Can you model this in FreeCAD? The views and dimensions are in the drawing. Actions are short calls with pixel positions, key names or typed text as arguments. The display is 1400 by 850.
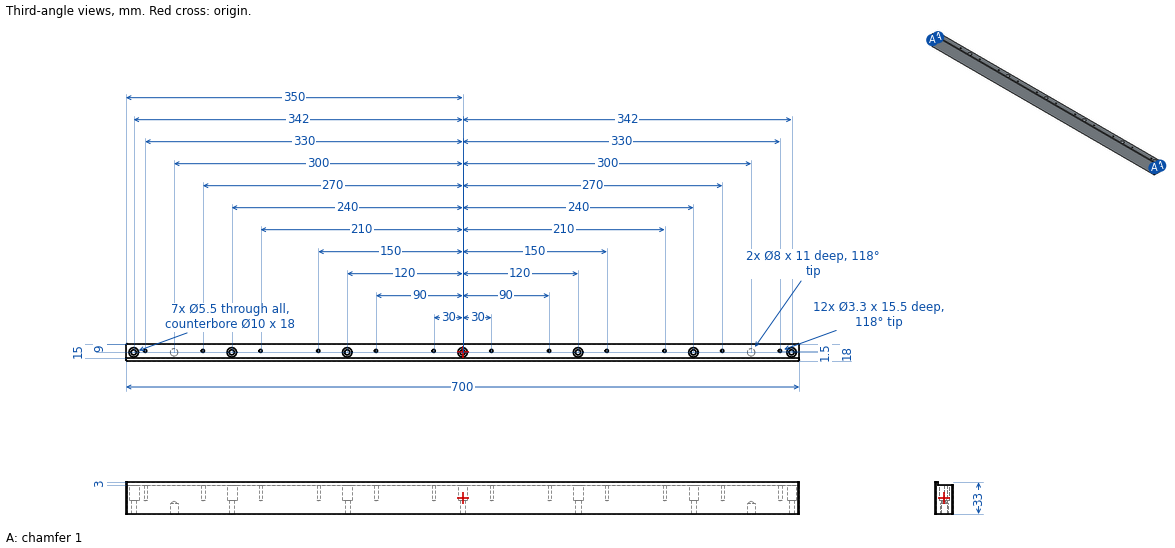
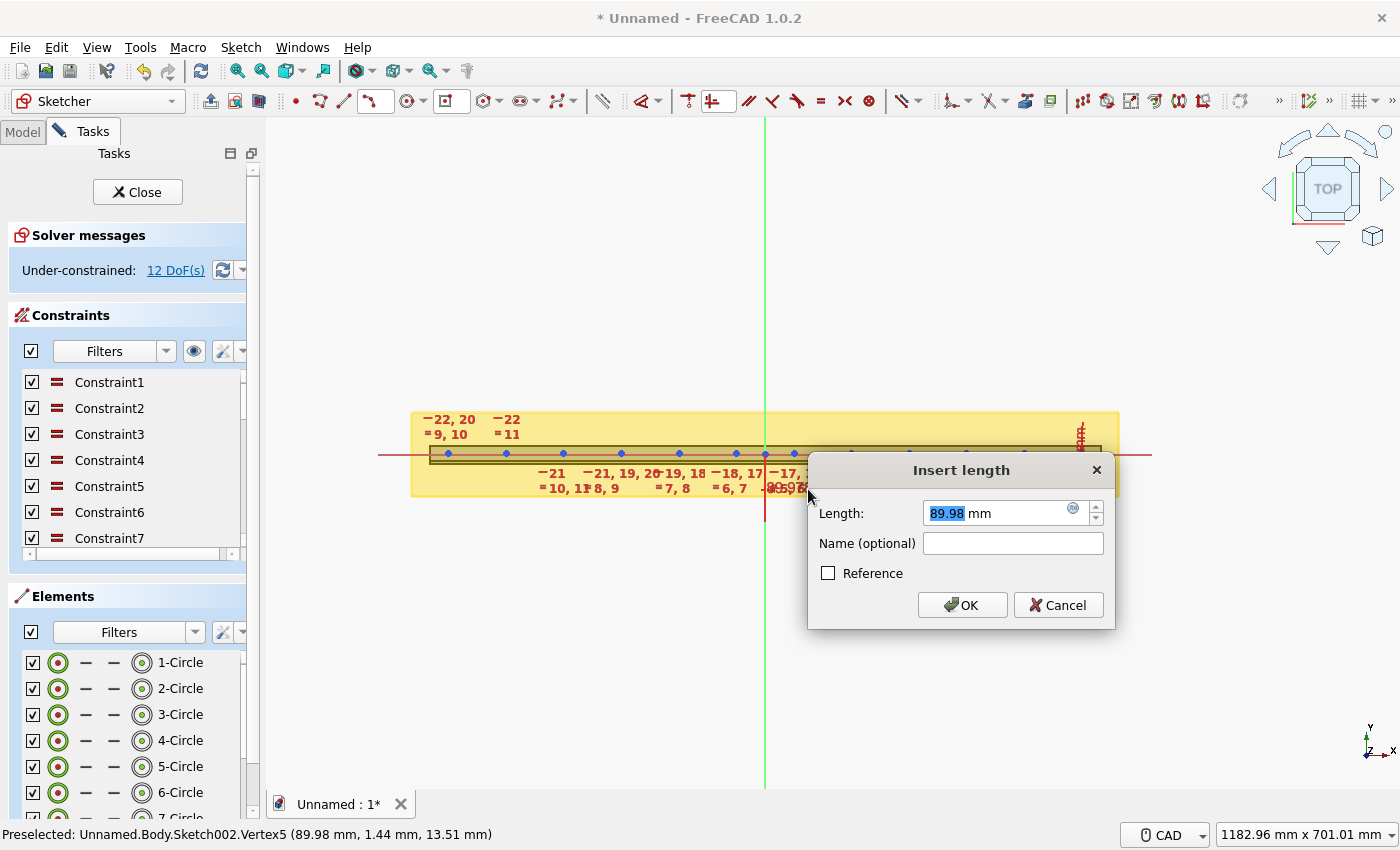
text(90)
key(Return)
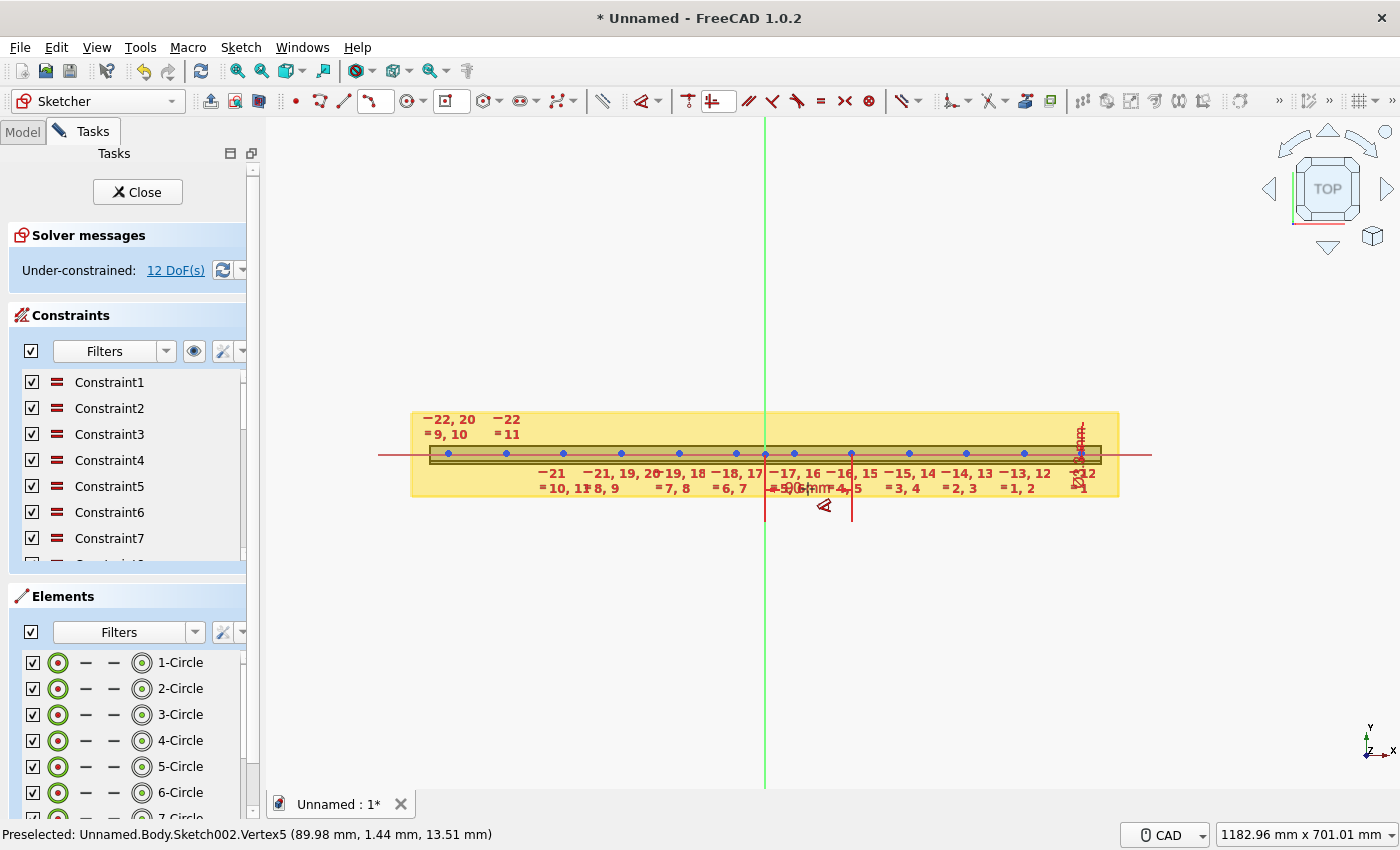
scroll(794, 453, up, 2)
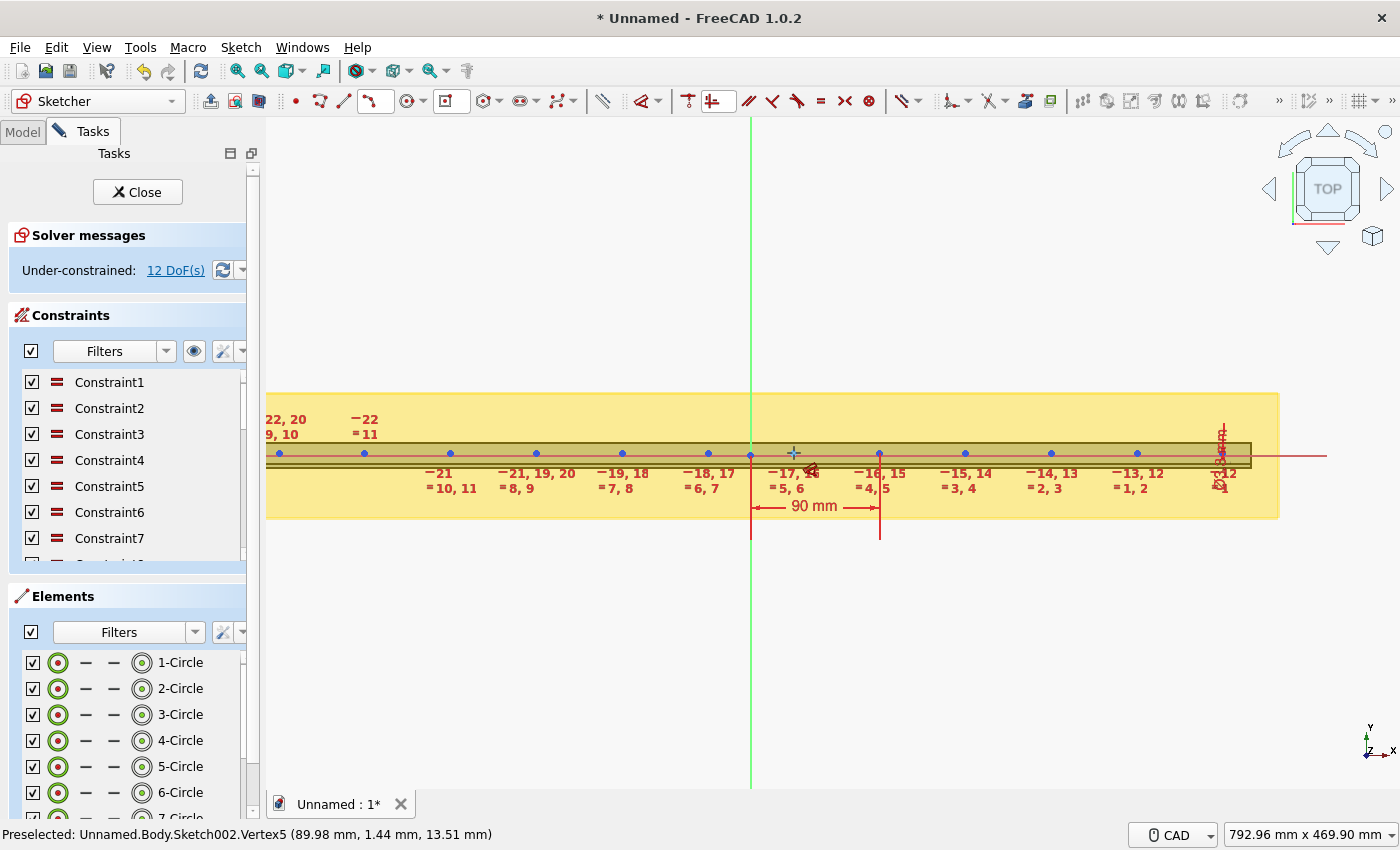
click(794, 453)
click(772, 419)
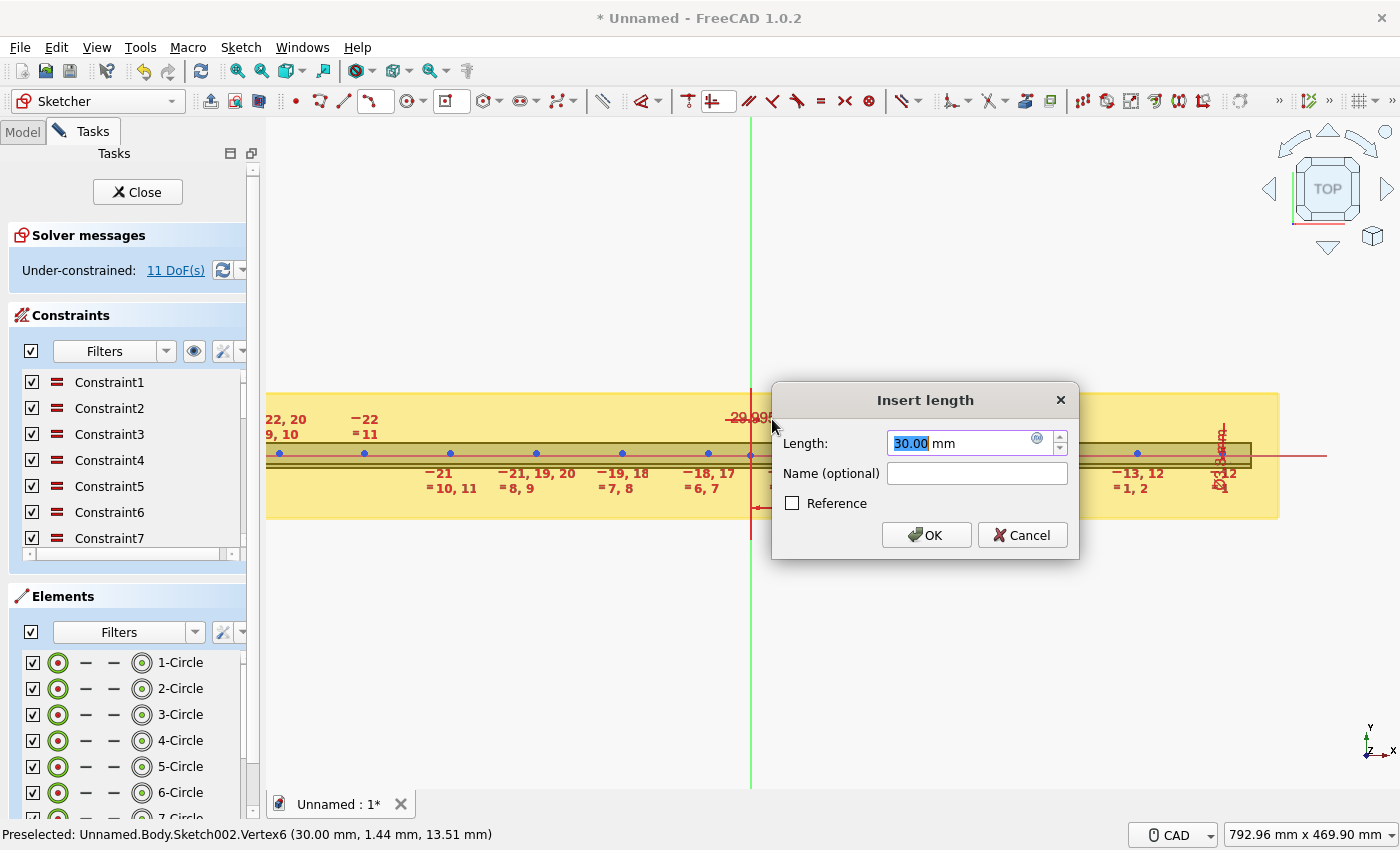
text(30)
key(Return)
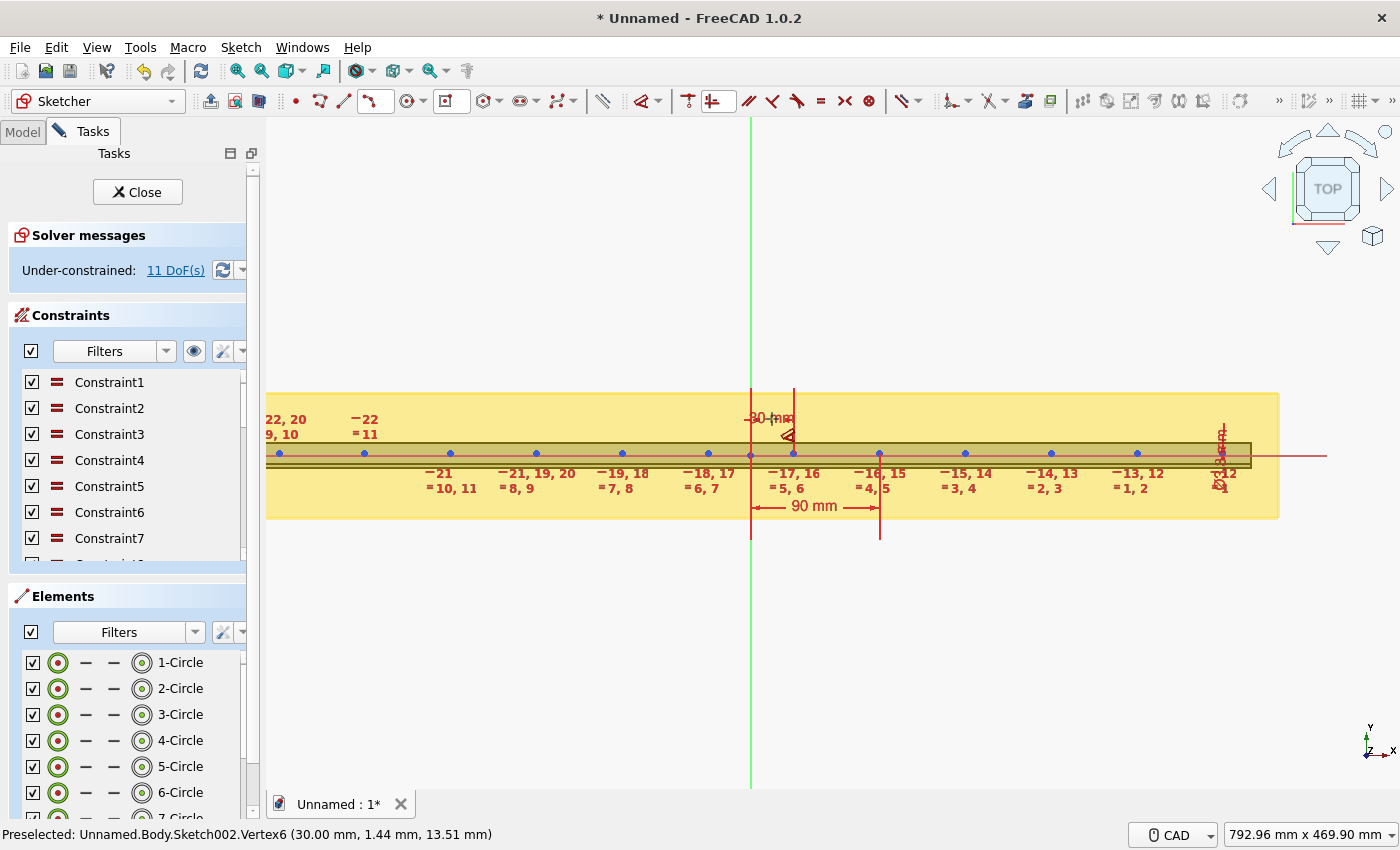
click(708, 453)
click(729, 490)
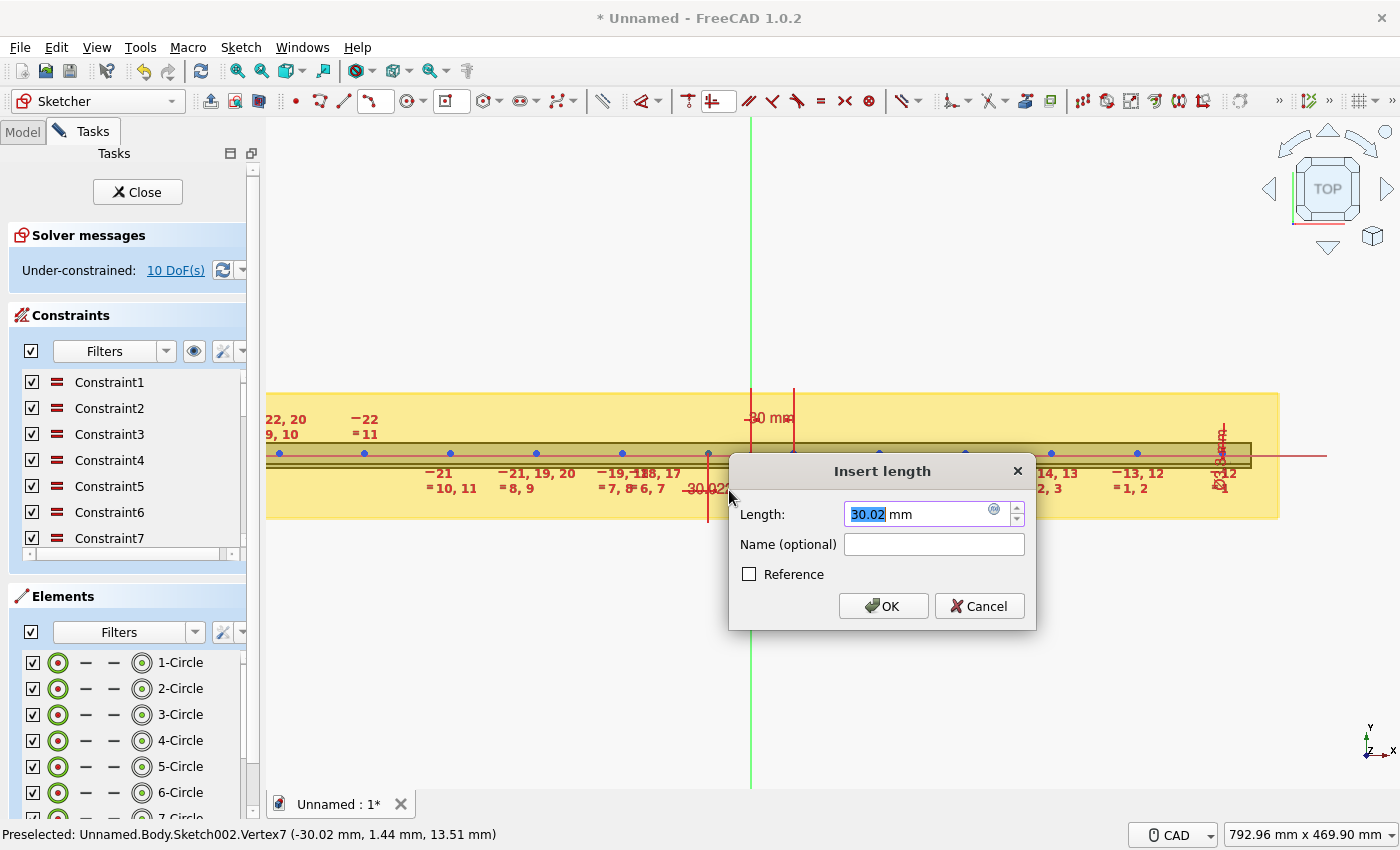
text(30)
key(Return)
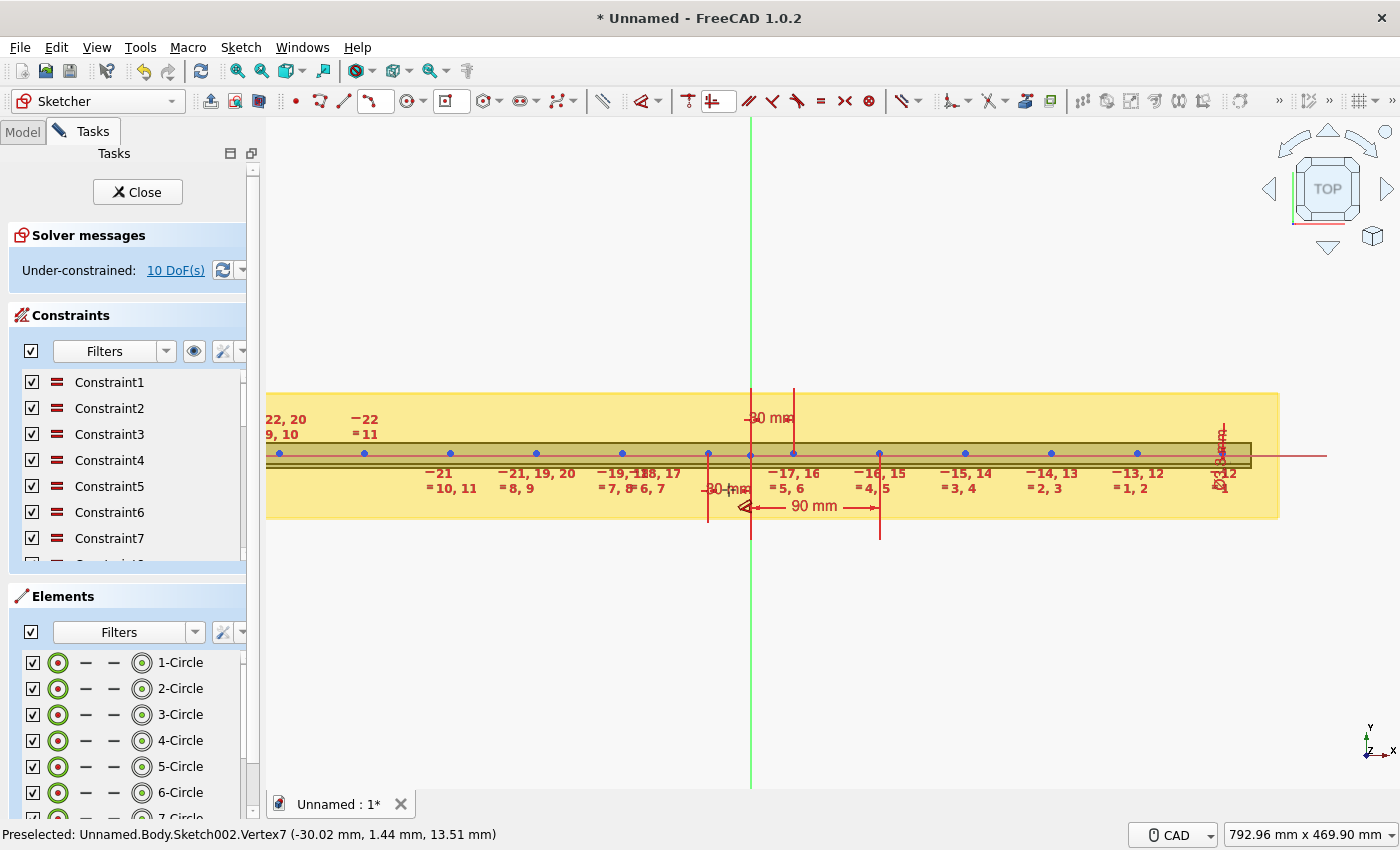
click(622, 453)
click(657, 490)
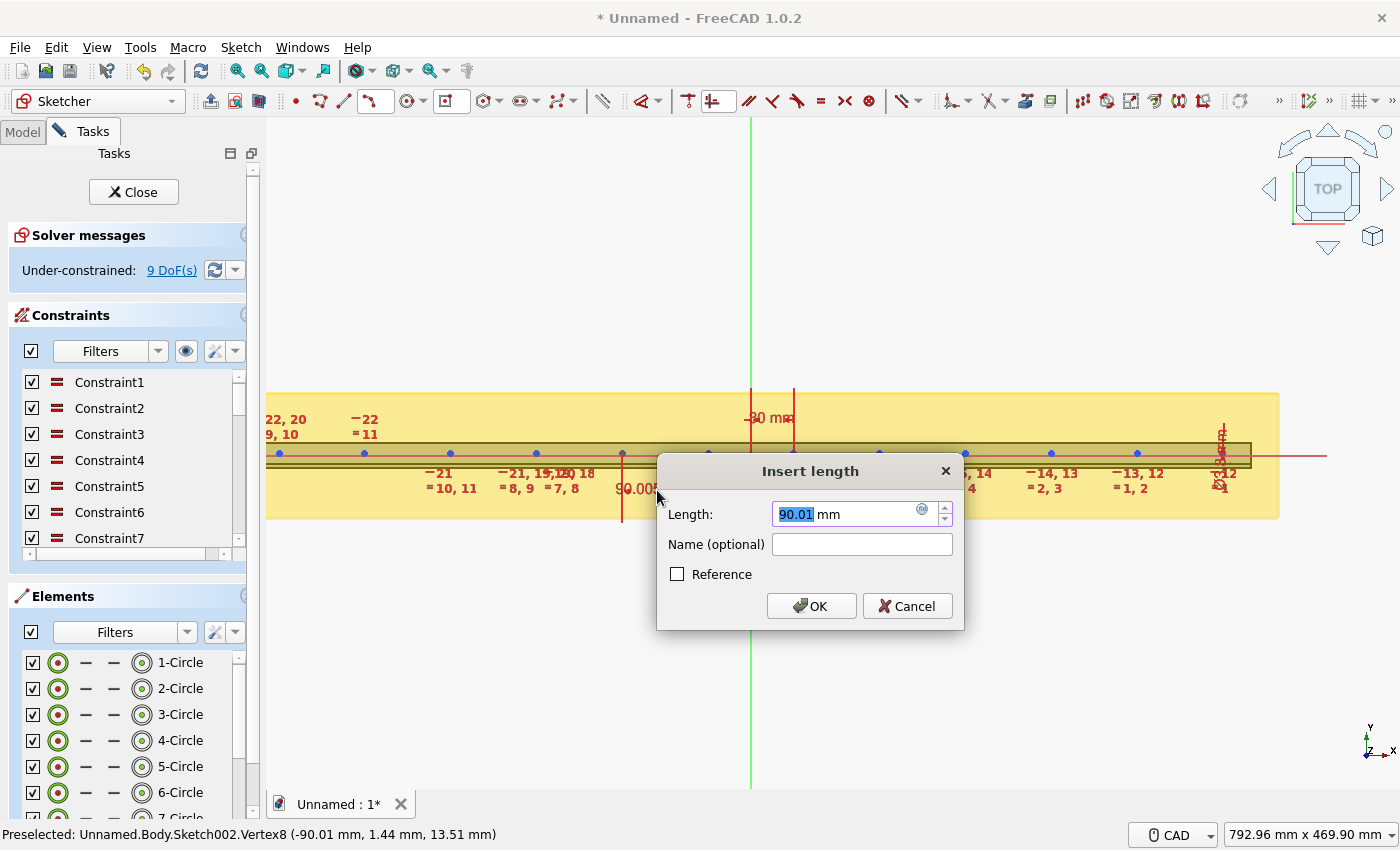
text(90)
key(Return)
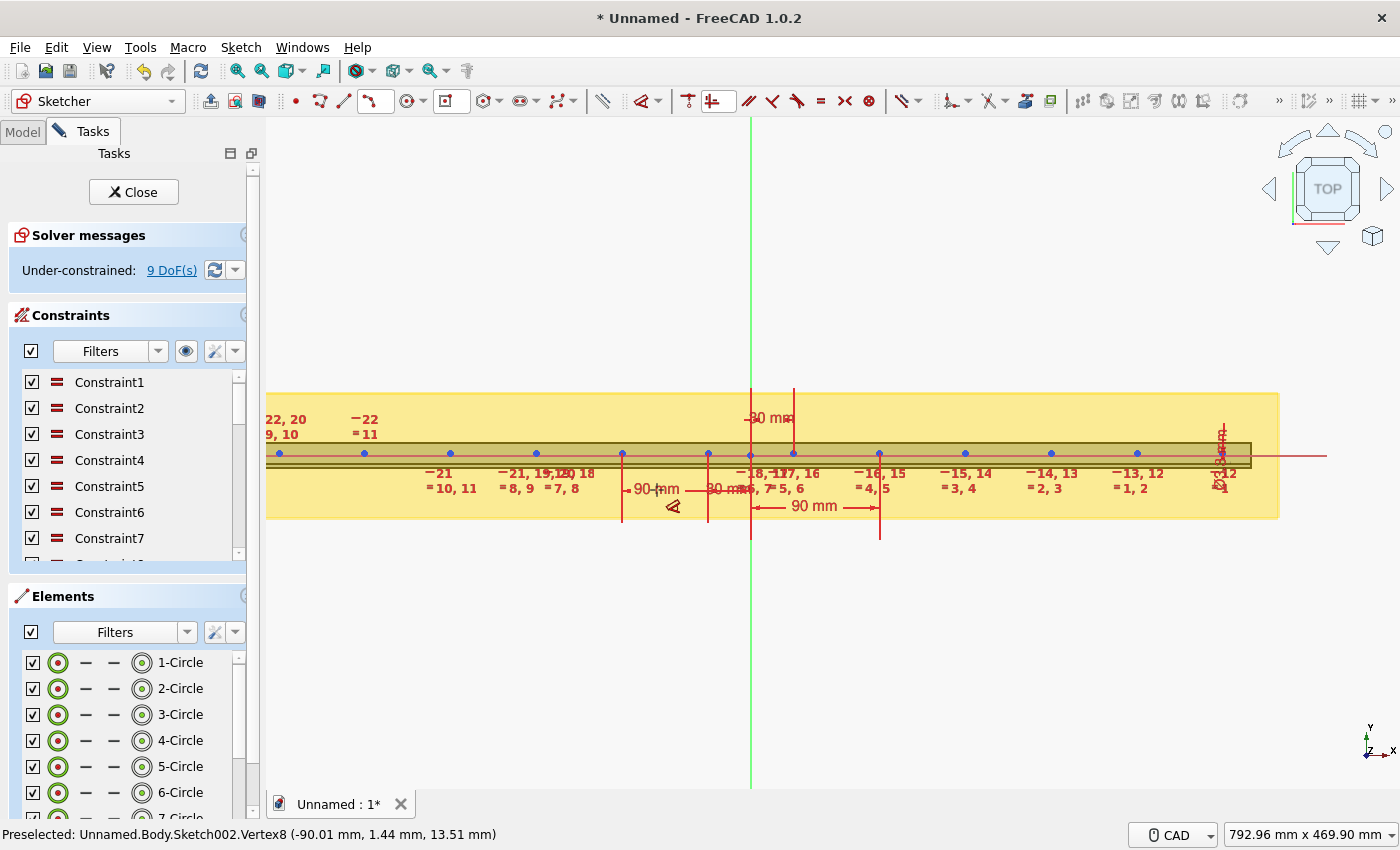
click(1223, 453)
click(987, 490)